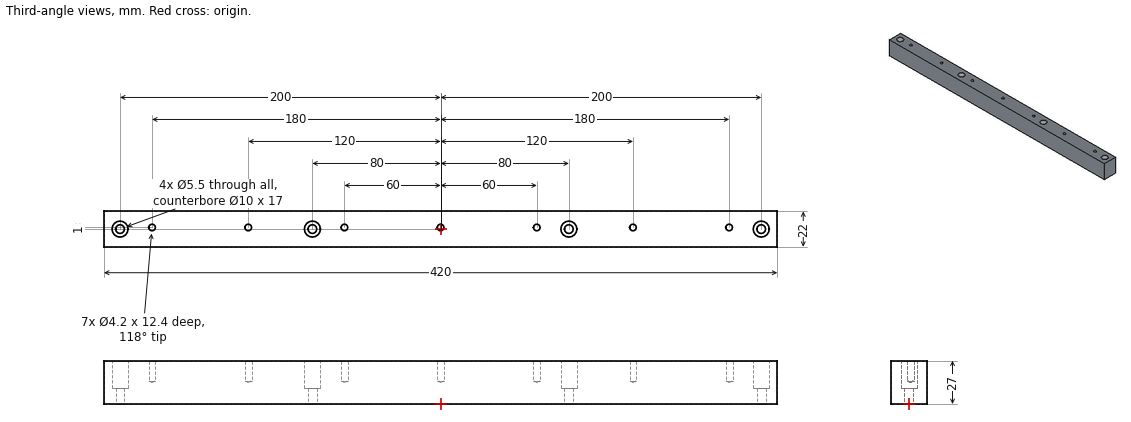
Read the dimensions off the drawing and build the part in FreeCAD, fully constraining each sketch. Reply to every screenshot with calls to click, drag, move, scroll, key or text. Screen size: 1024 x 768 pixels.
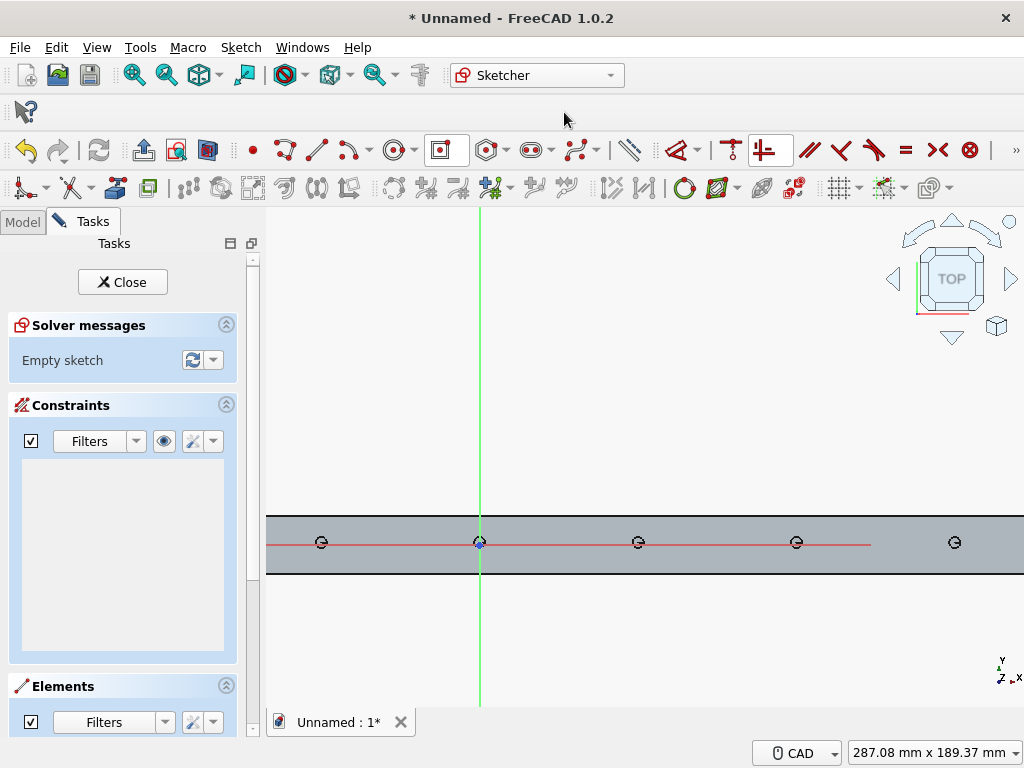
scroll(633, 406, down, 5)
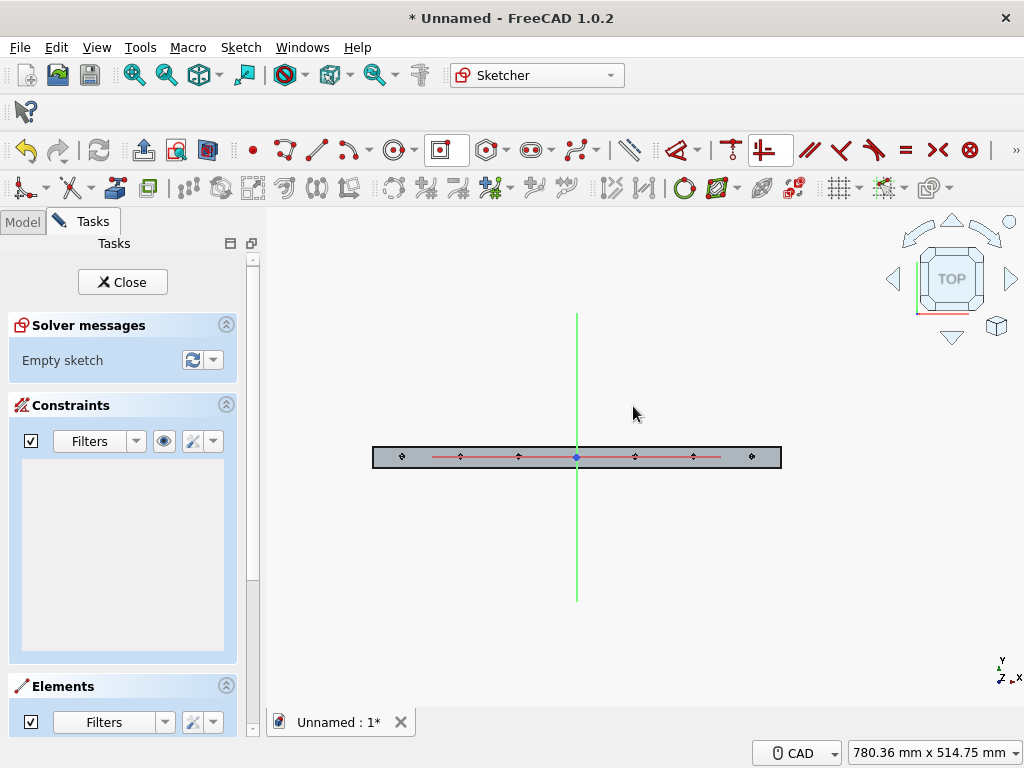
key(g)
key(c)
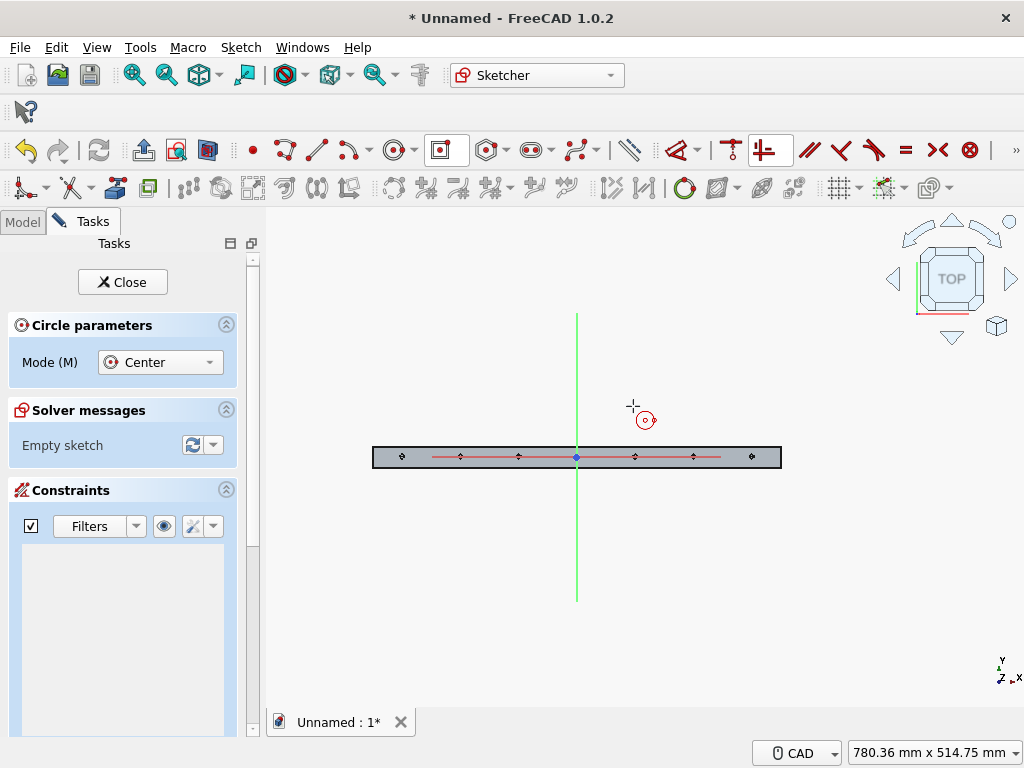
scroll(383, 457, up, 11)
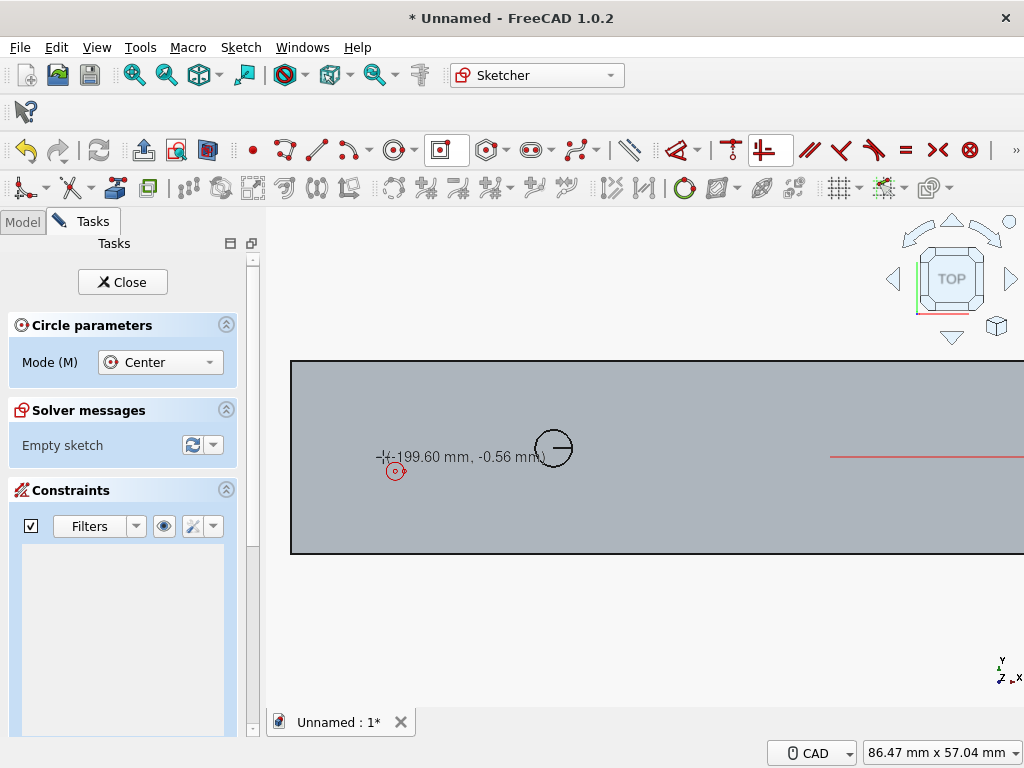
scroll(383, 457, down, 11)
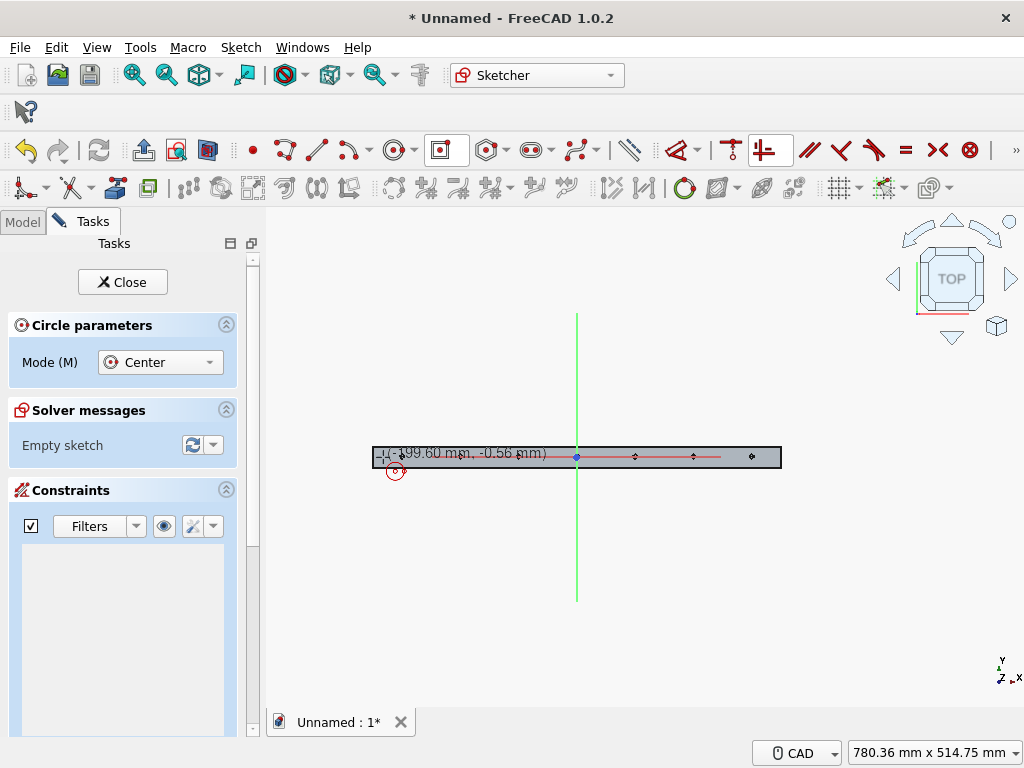
click(383, 457)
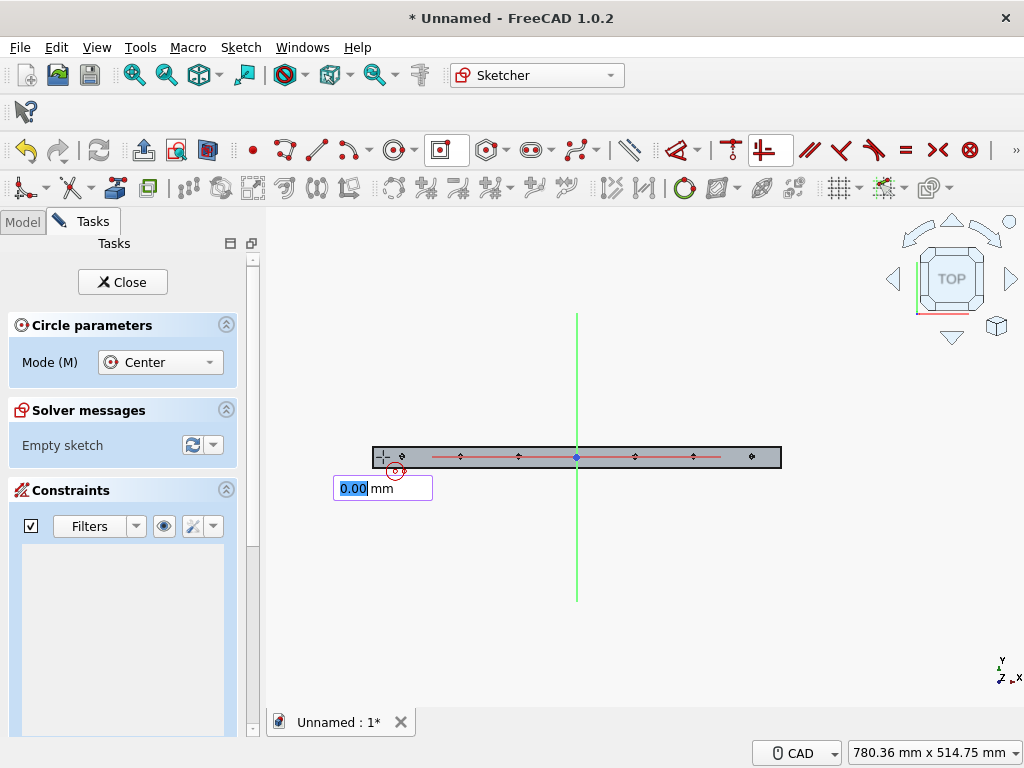
scroll(384, 455, up, 10)
move(380, 451)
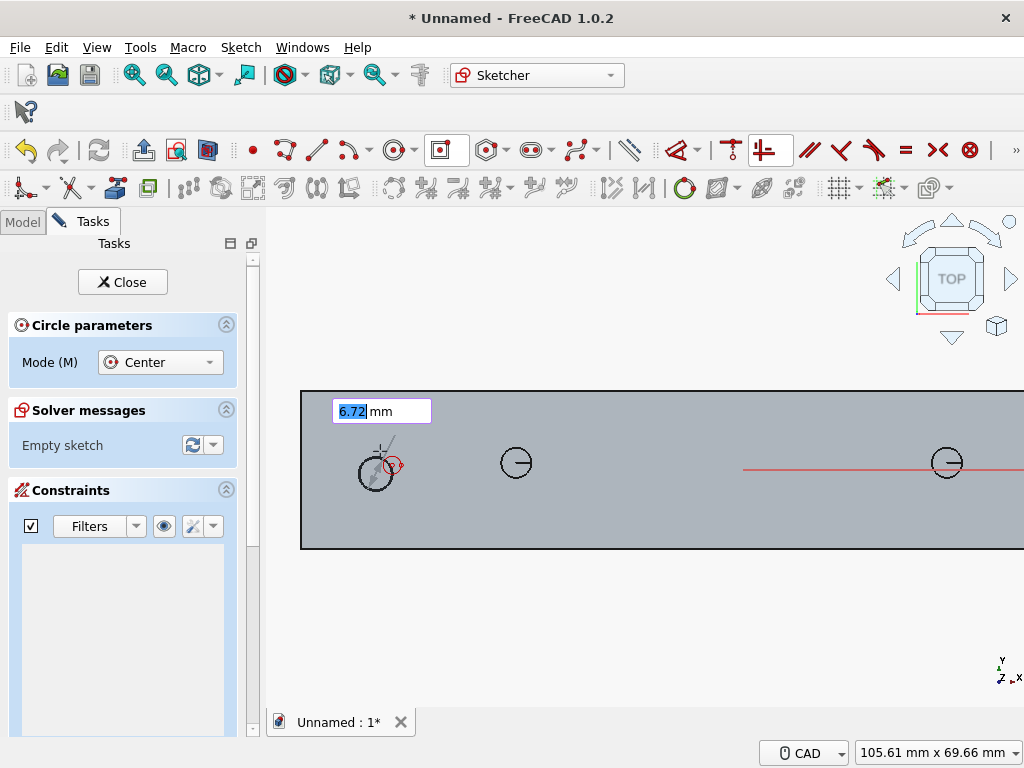
text(5.5)
key(Return)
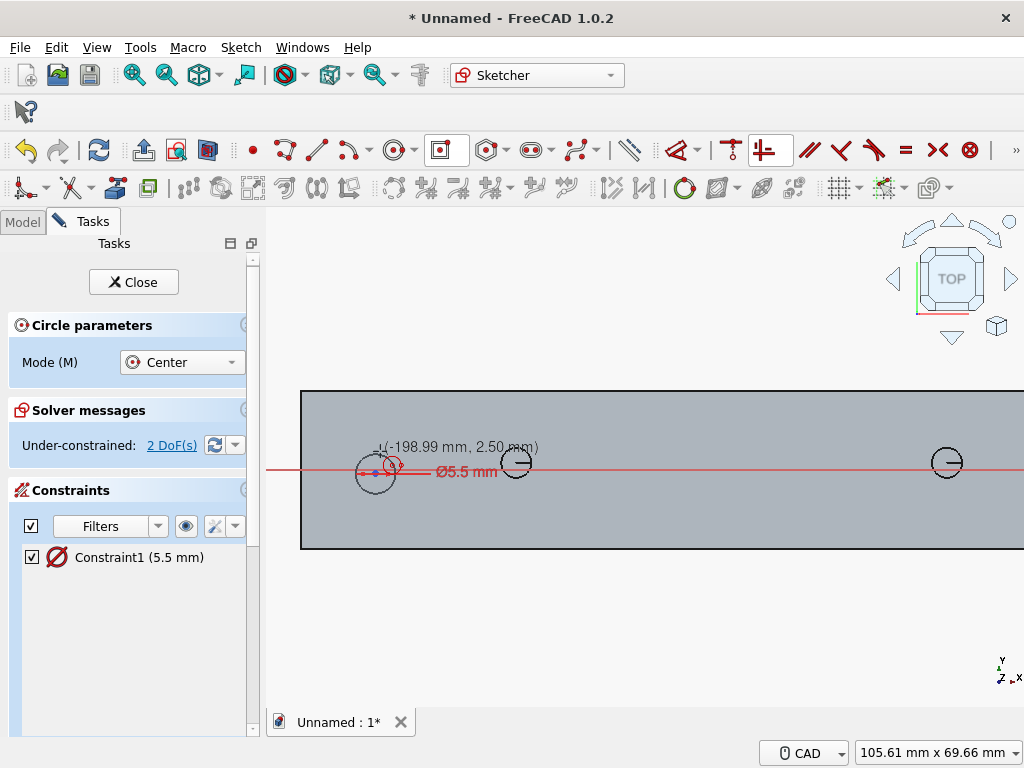
scroll(384, 455, down, 10)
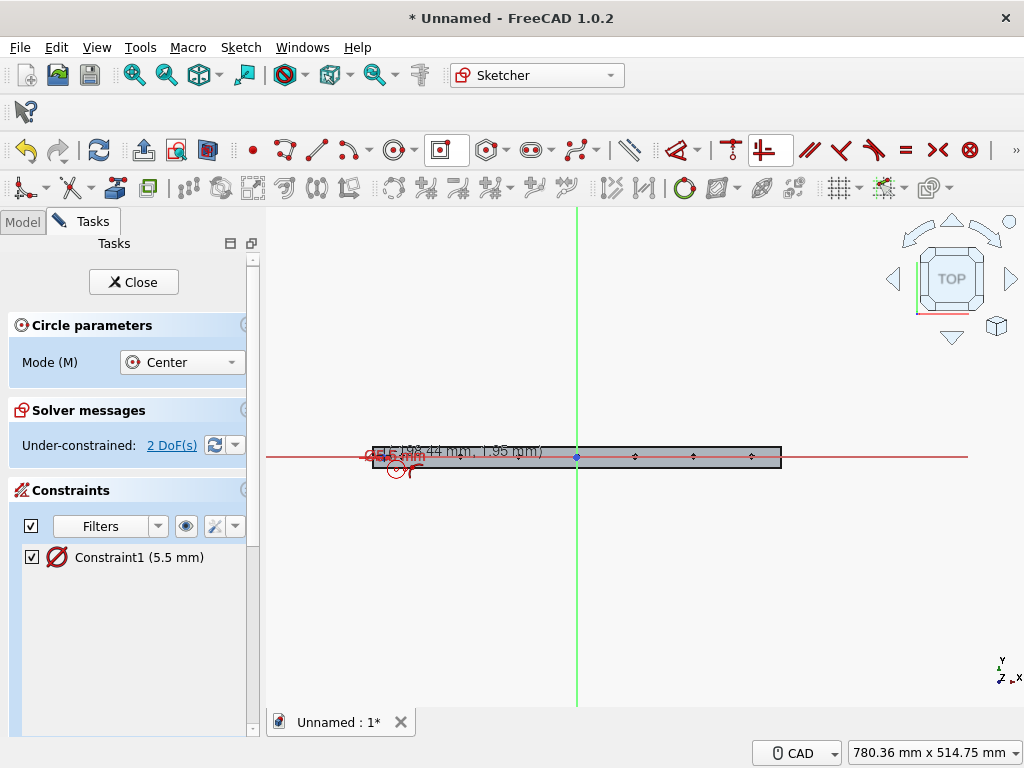
scroll(499, 457, up, 11)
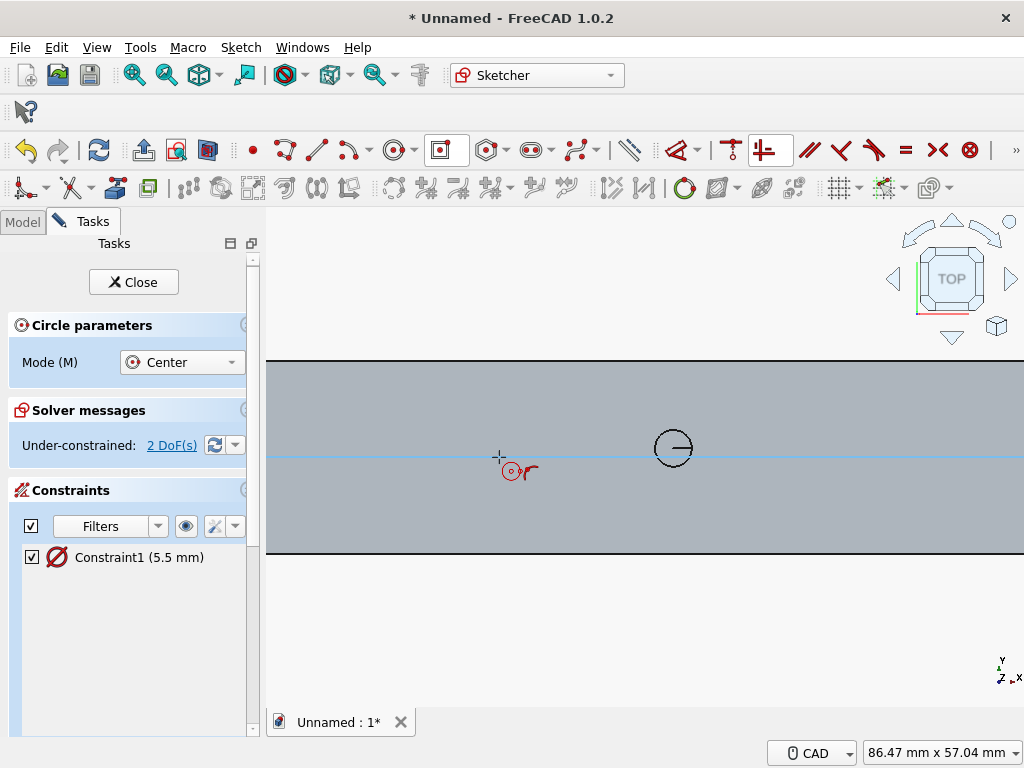
scroll(499, 457, down, 11)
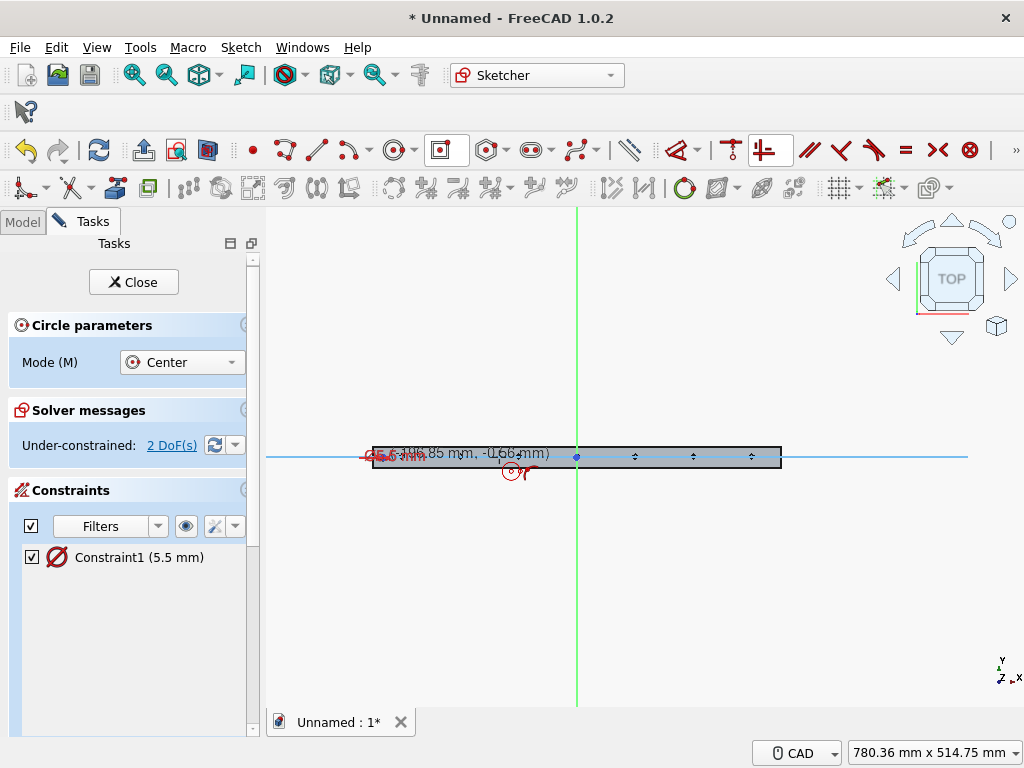
click(499, 457)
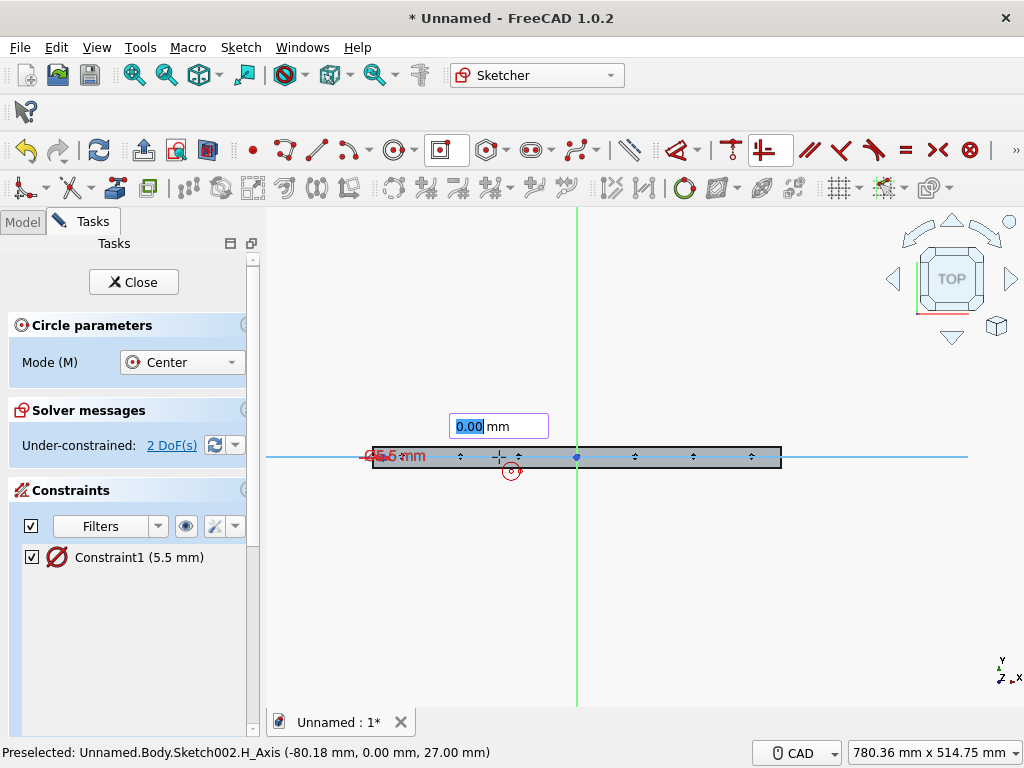
scroll(500, 455, up, 10)
move(499, 451)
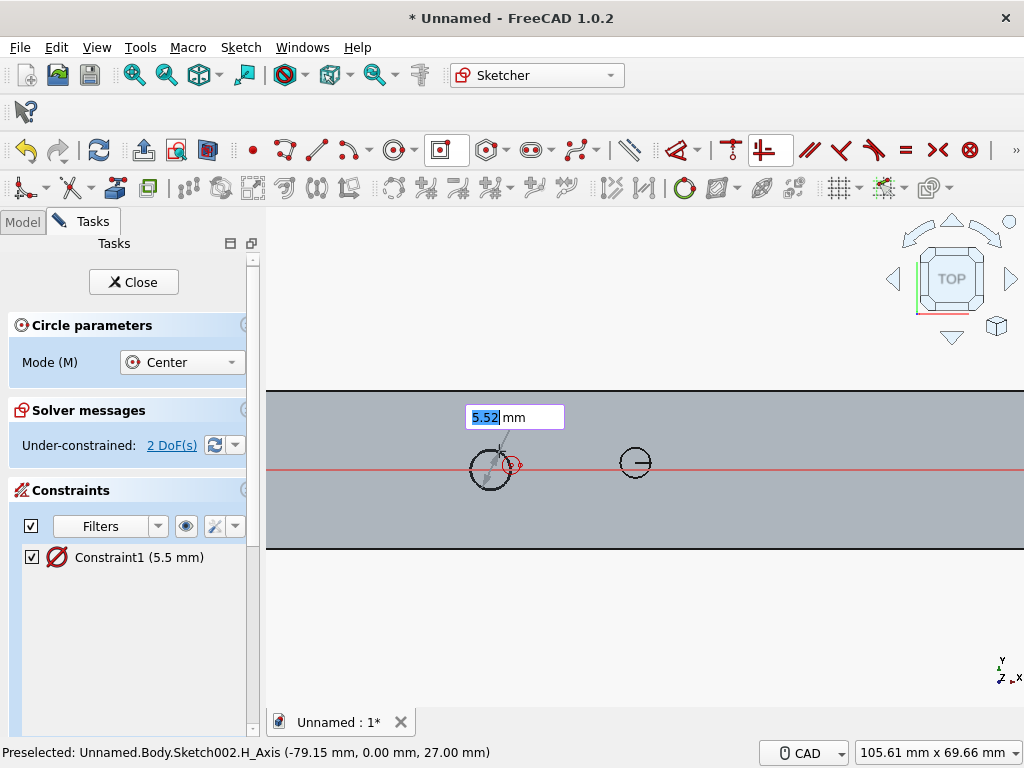
text(5.5)
key(Return)